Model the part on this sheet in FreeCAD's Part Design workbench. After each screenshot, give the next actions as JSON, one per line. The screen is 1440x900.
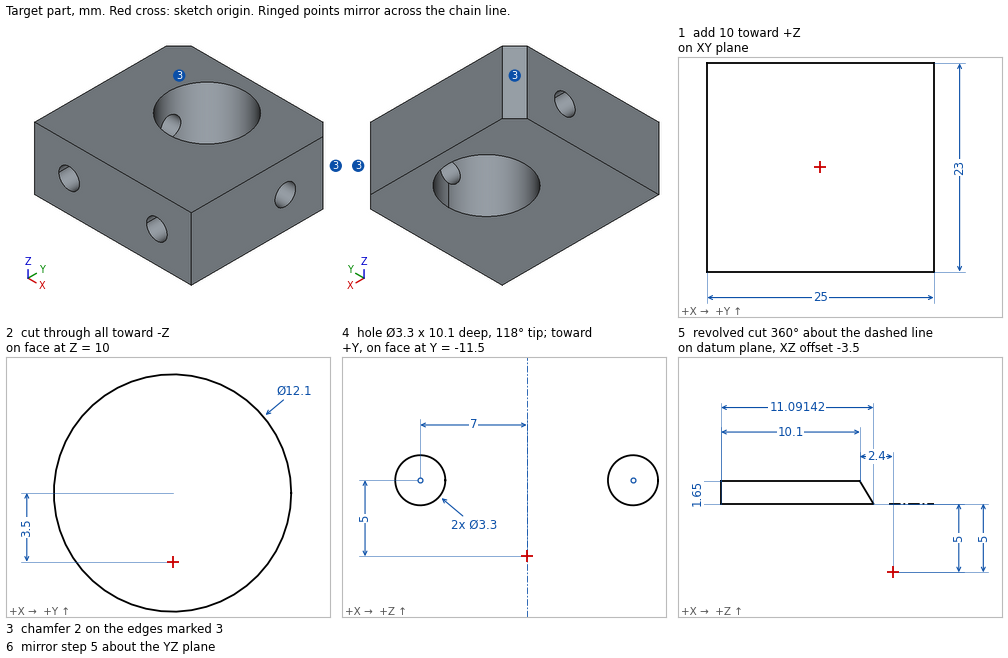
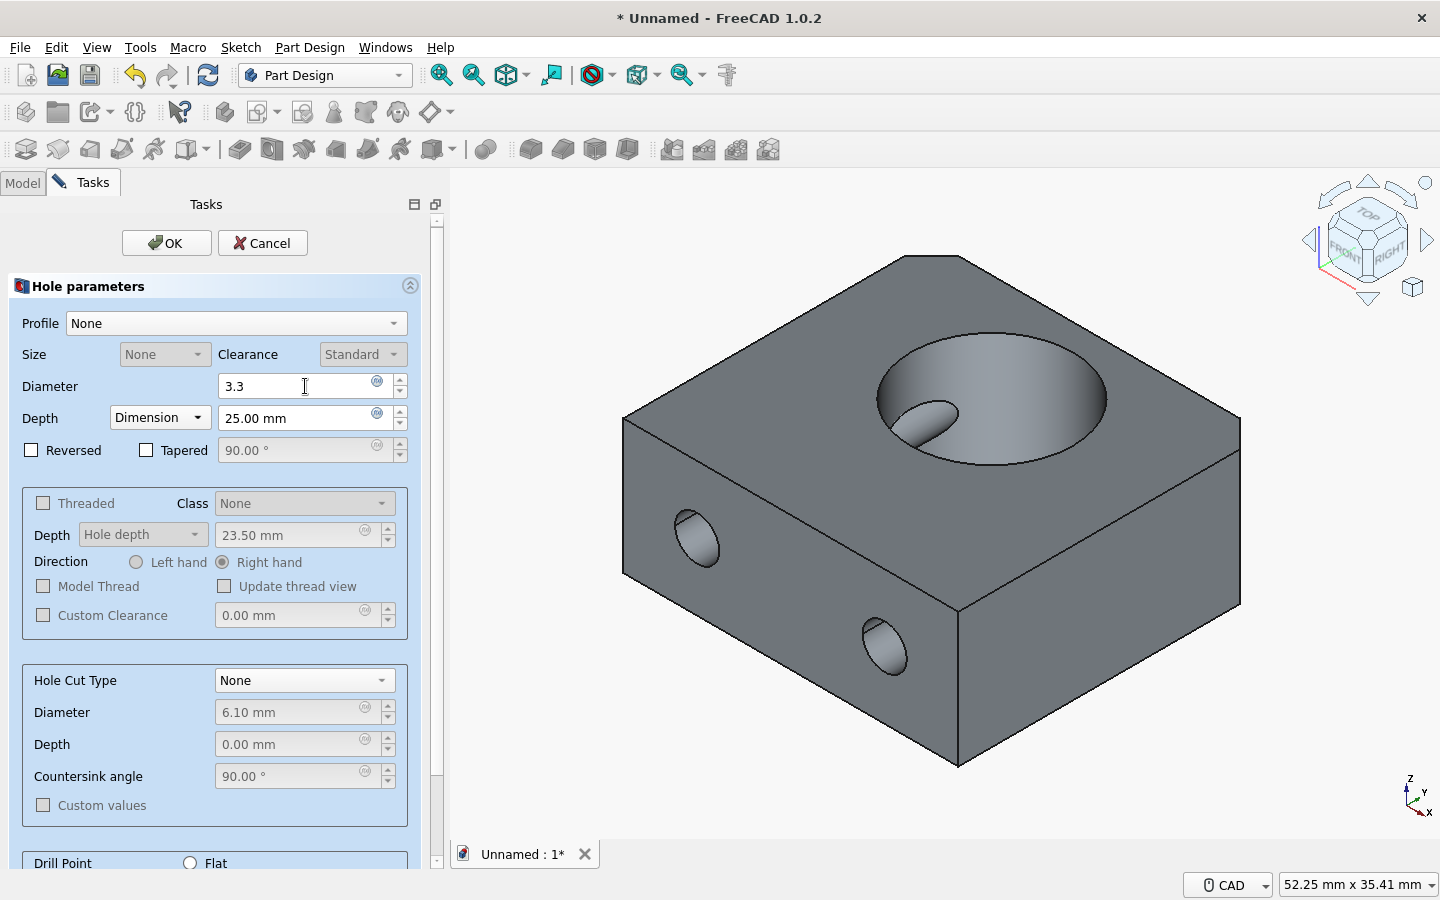
{"action": "triple_click", "coordinate": [305, 418]}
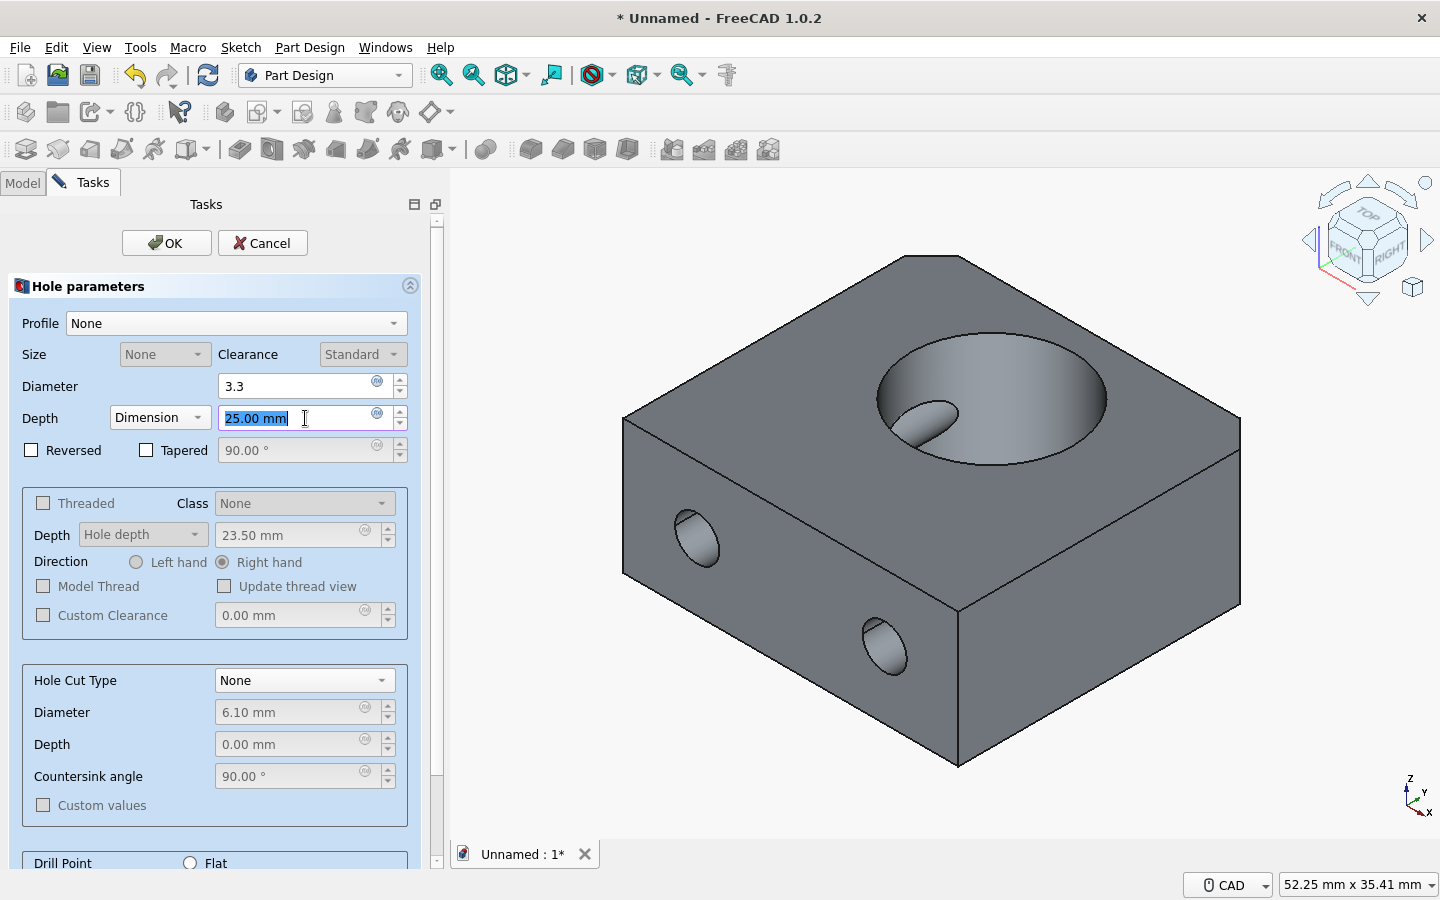
{"action": "type", "text": "10.1"}
{"action": "key", "text": "Tab"}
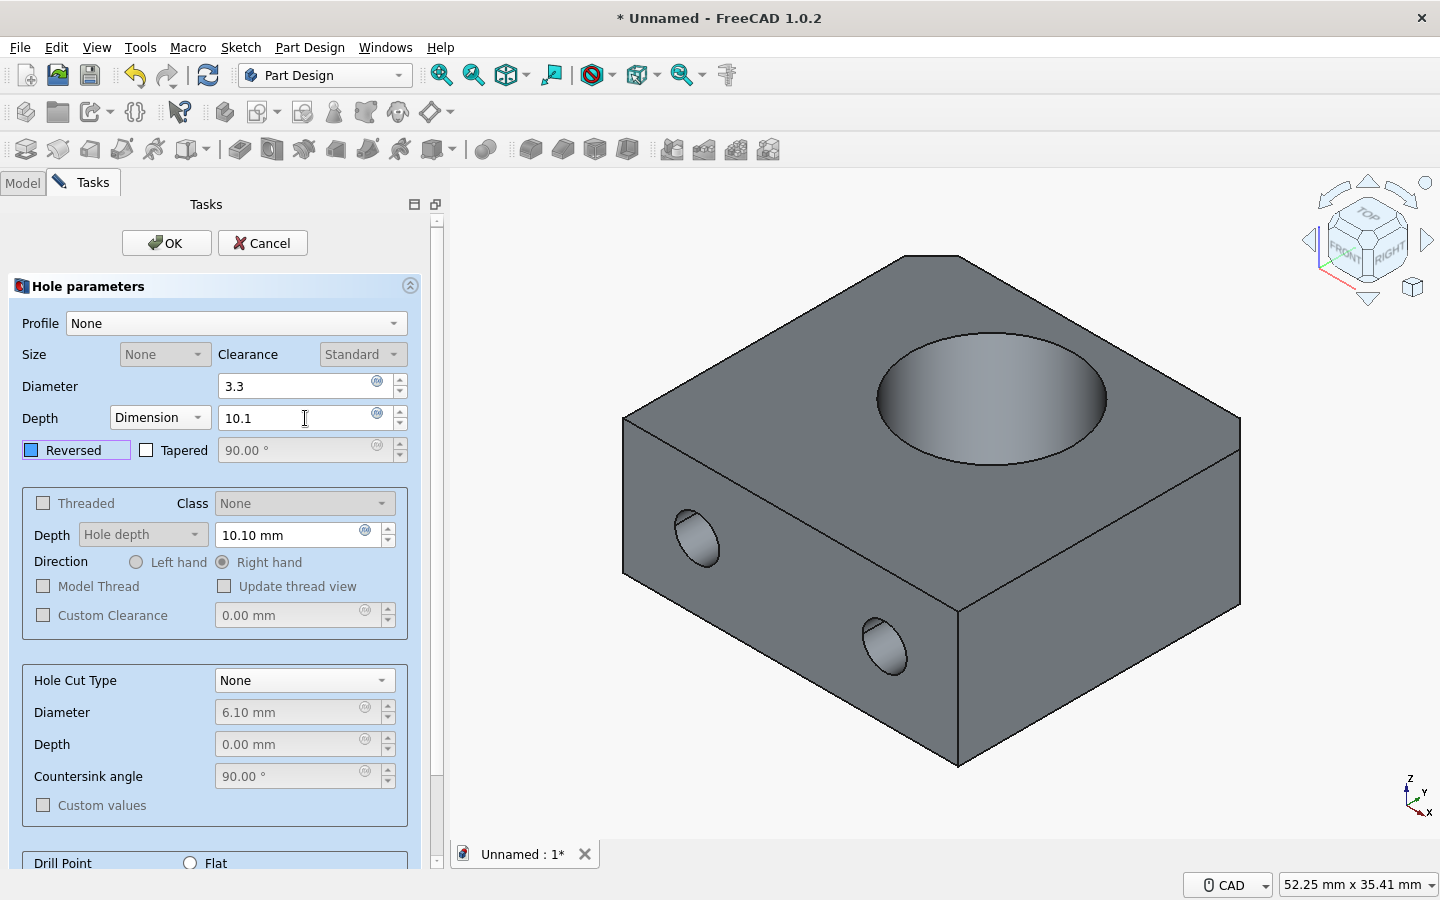
{"action": "left_click", "coordinate": [167, 243]}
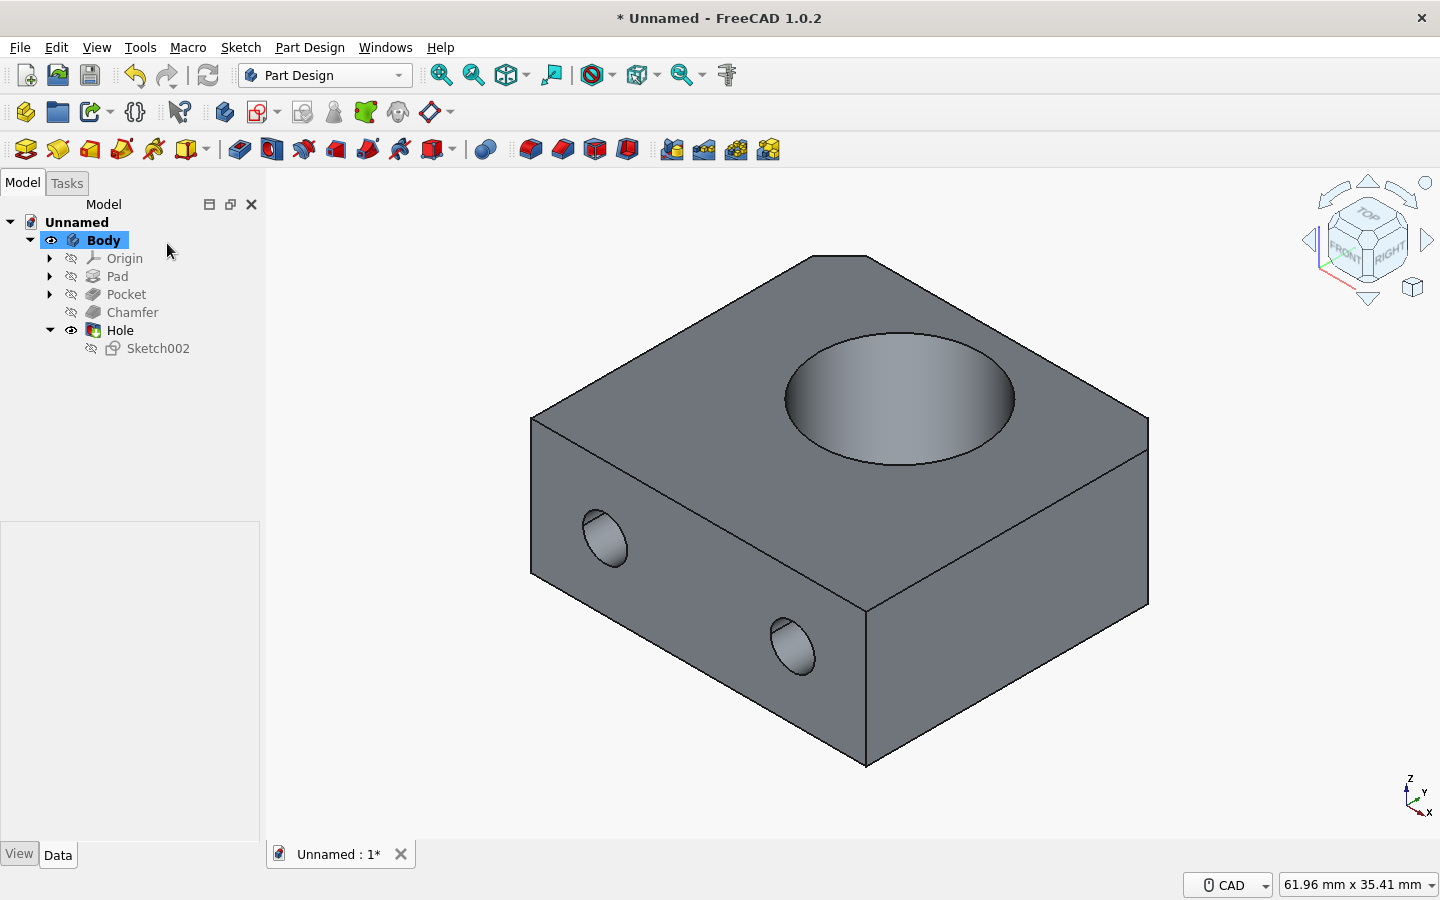
{"action": "left_click", "coordinate": [50, 258]}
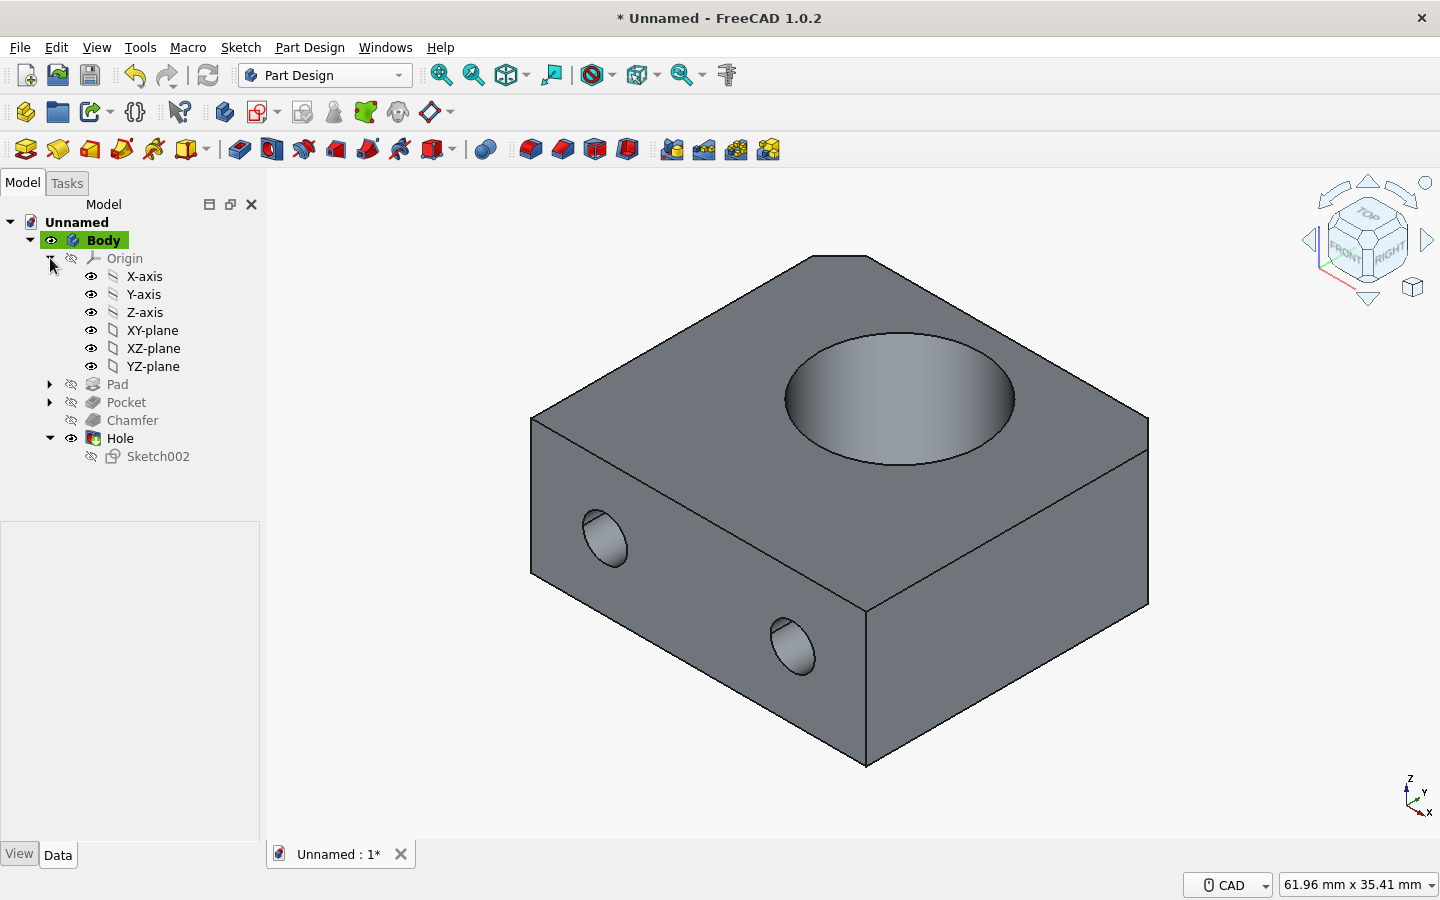
{"action": "left_click", "coordinate": [136, 348]}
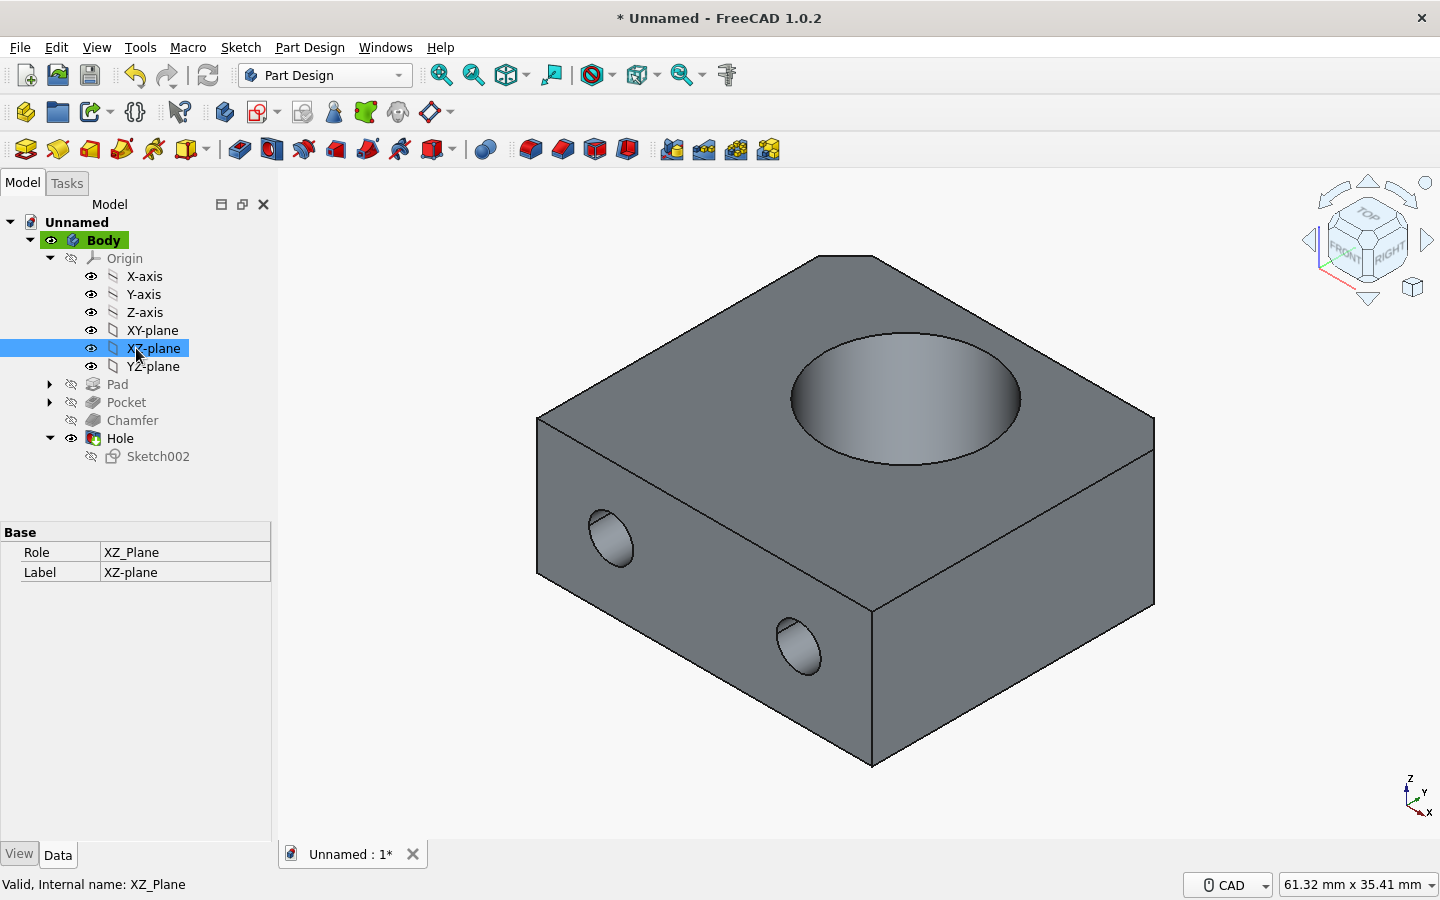
{"action": "left_click", "coordinate": [430, 112]}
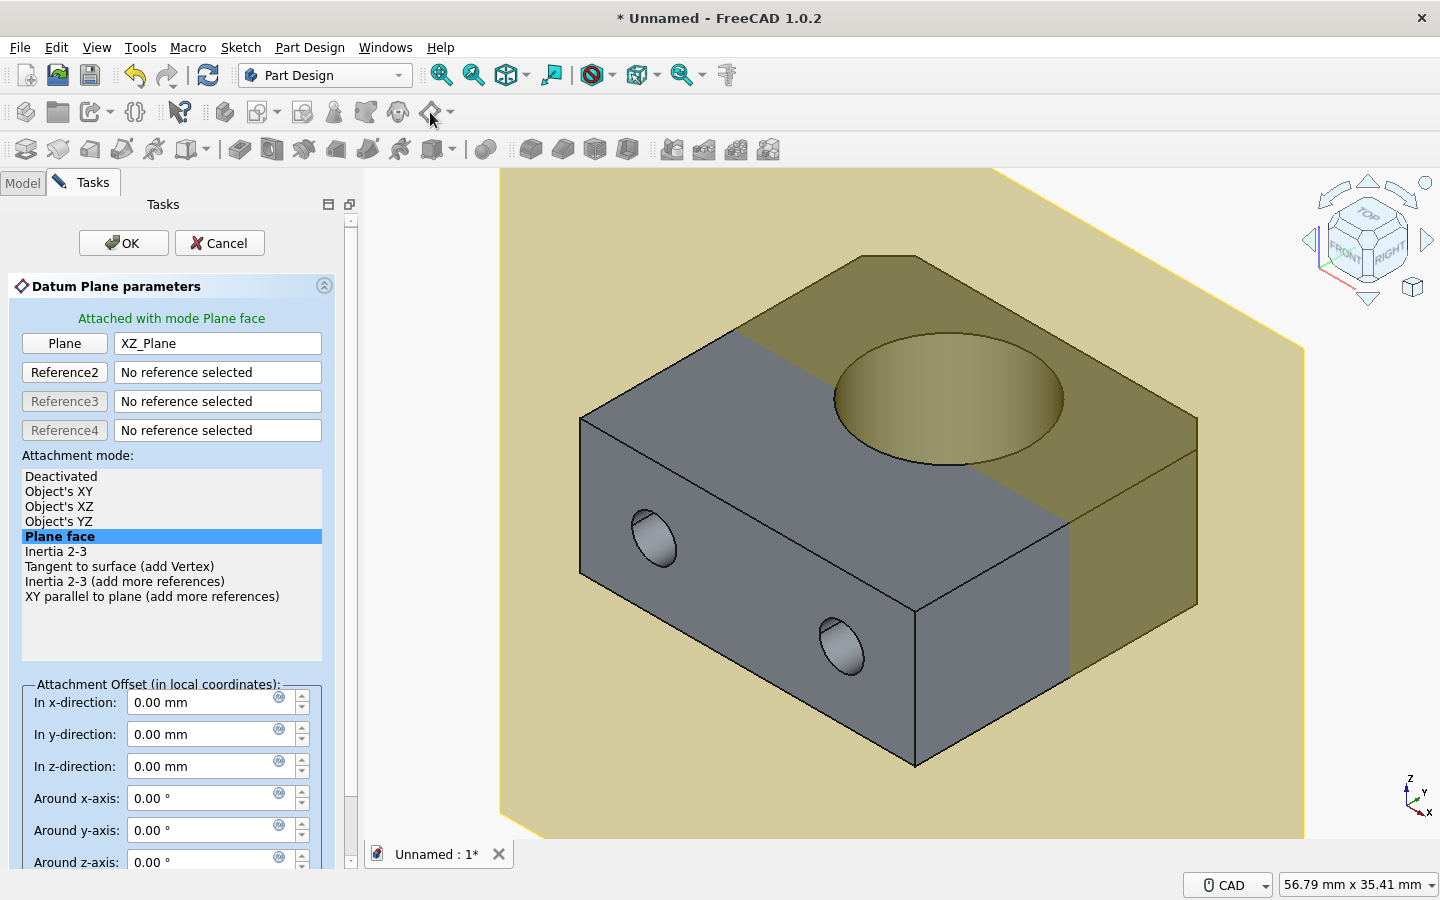
{"action": "triple_click", "coordinate": [210, 766]}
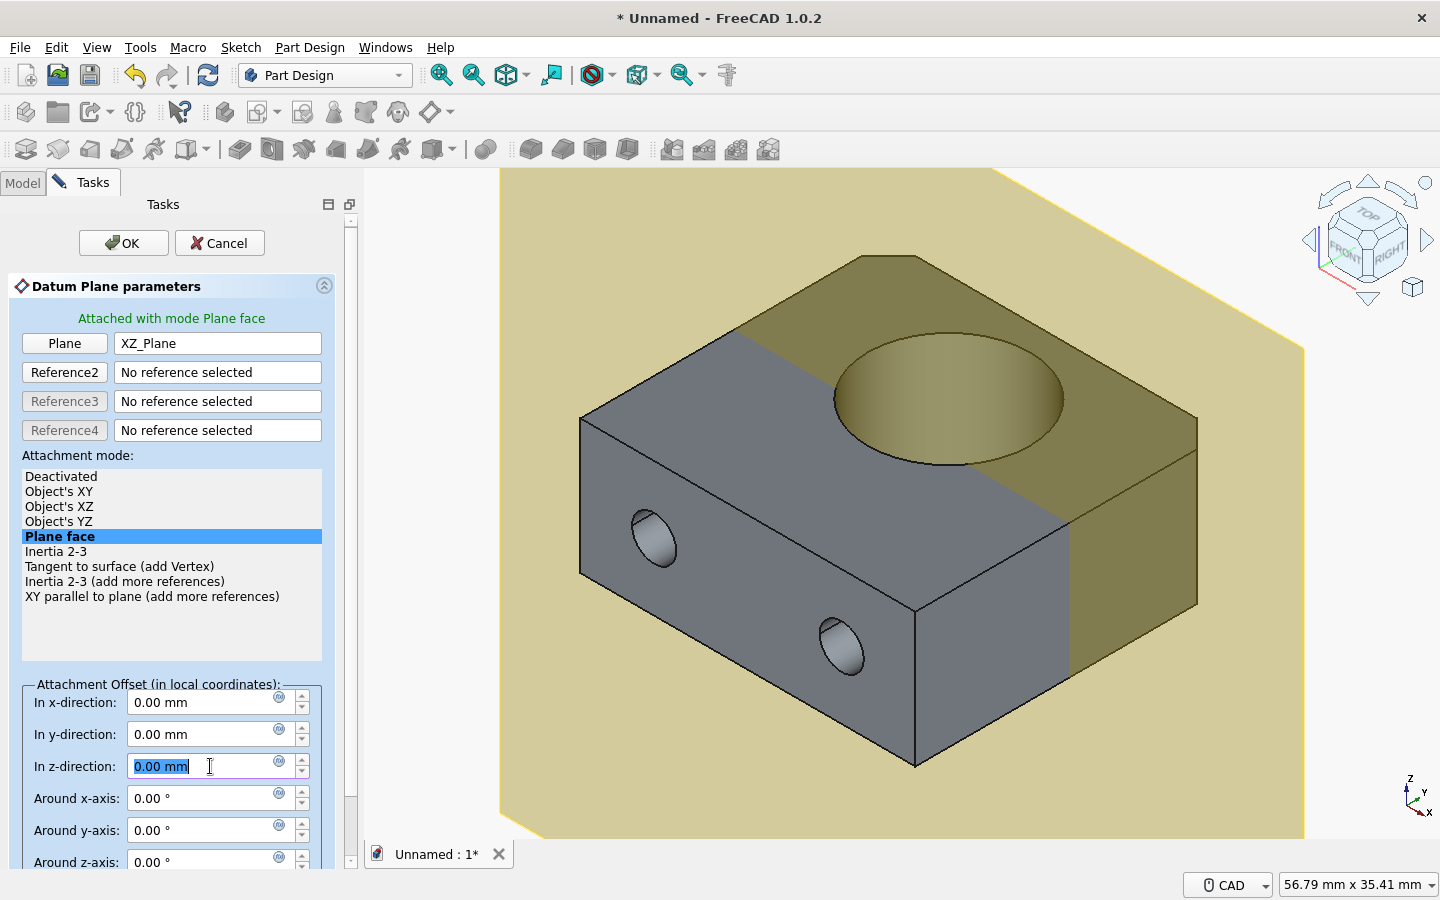
{"action": "type", "text": "-3.5"}
{"action": "key", "text": "Tab"}